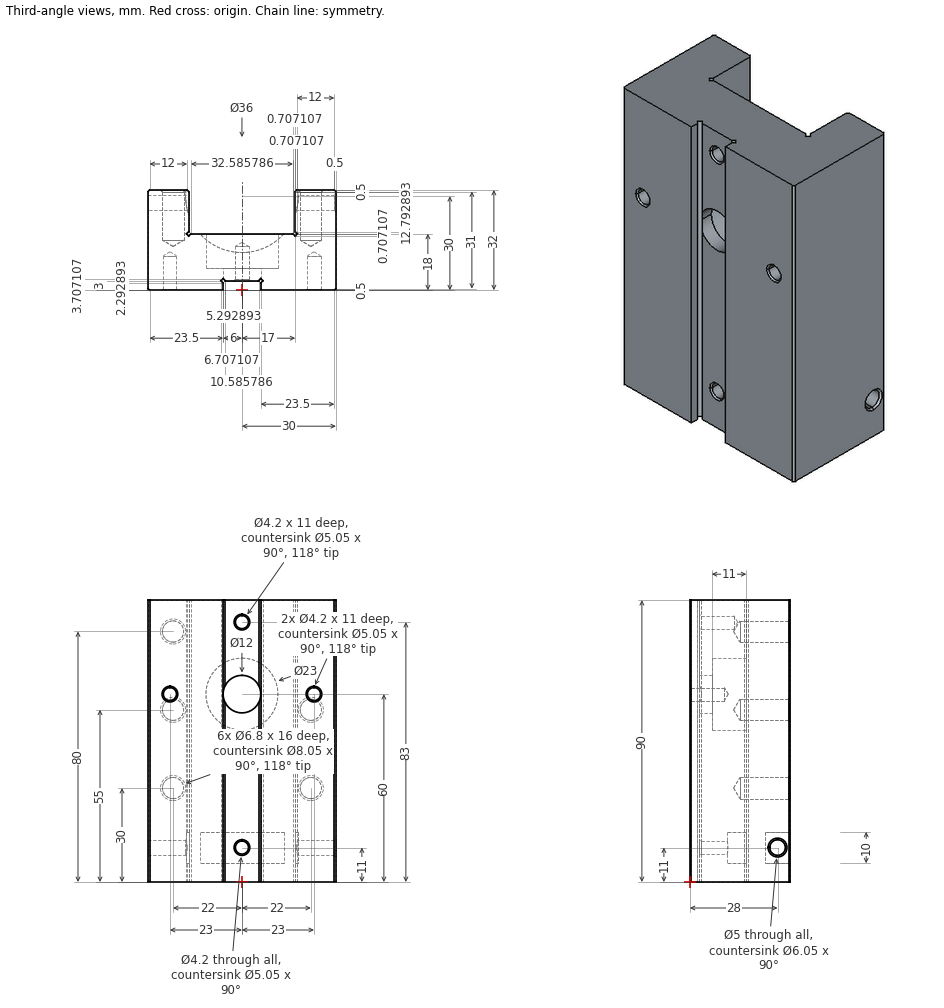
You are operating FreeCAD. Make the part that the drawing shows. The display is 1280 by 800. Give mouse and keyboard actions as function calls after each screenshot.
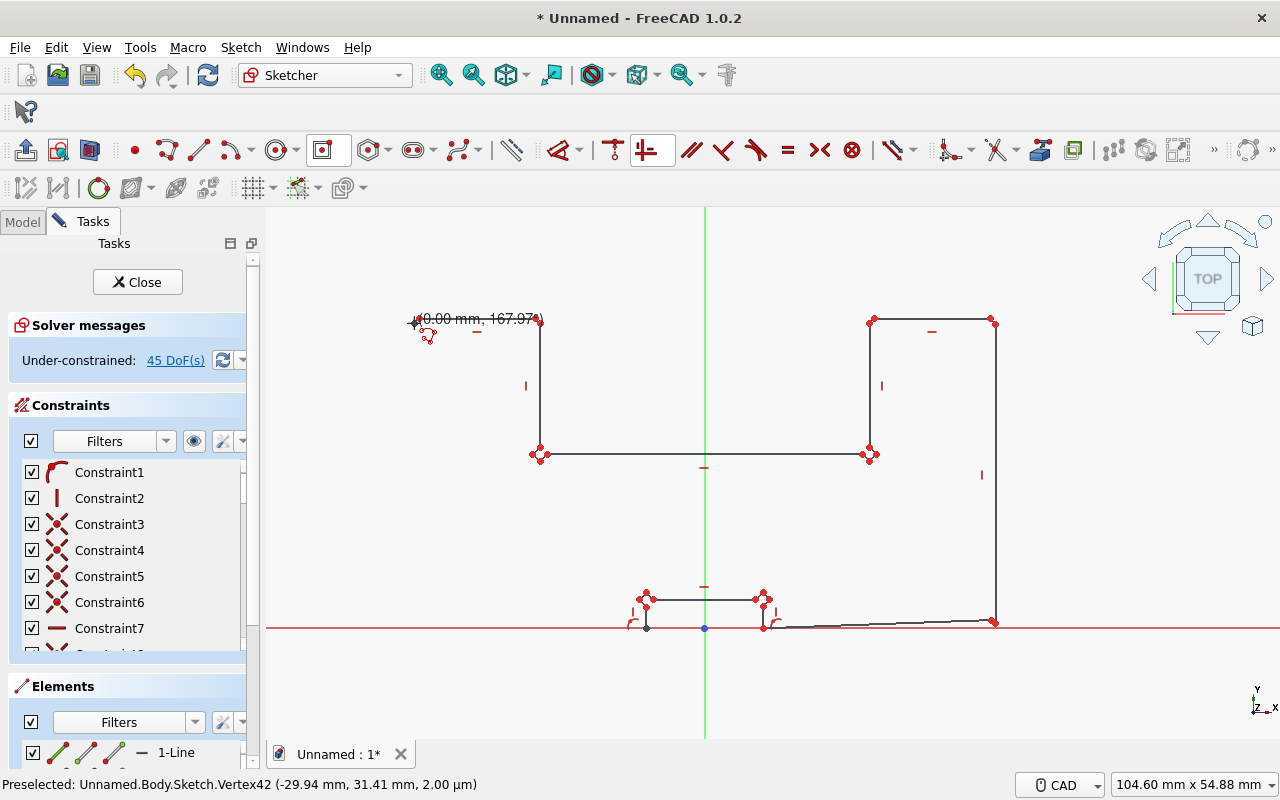
scroll(414, 623, up, 6)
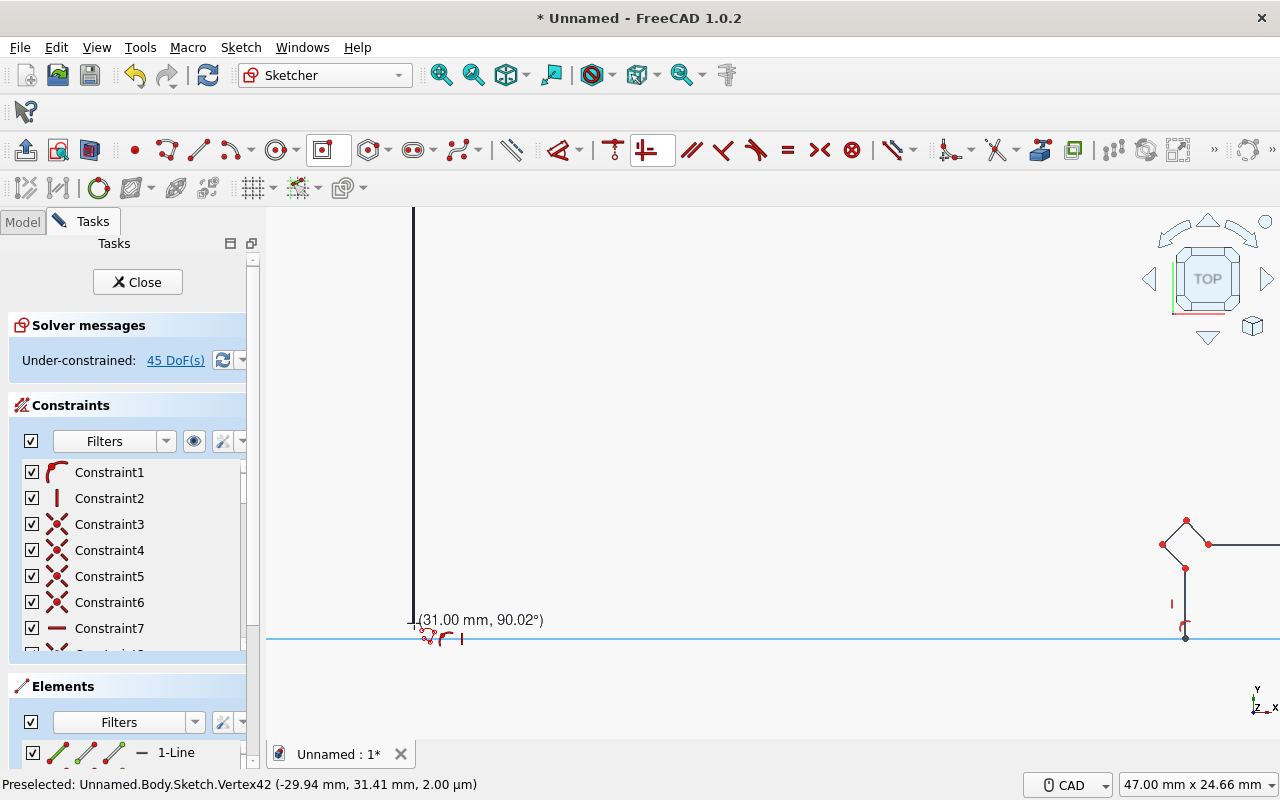
click(414, 623)
click(430, 630)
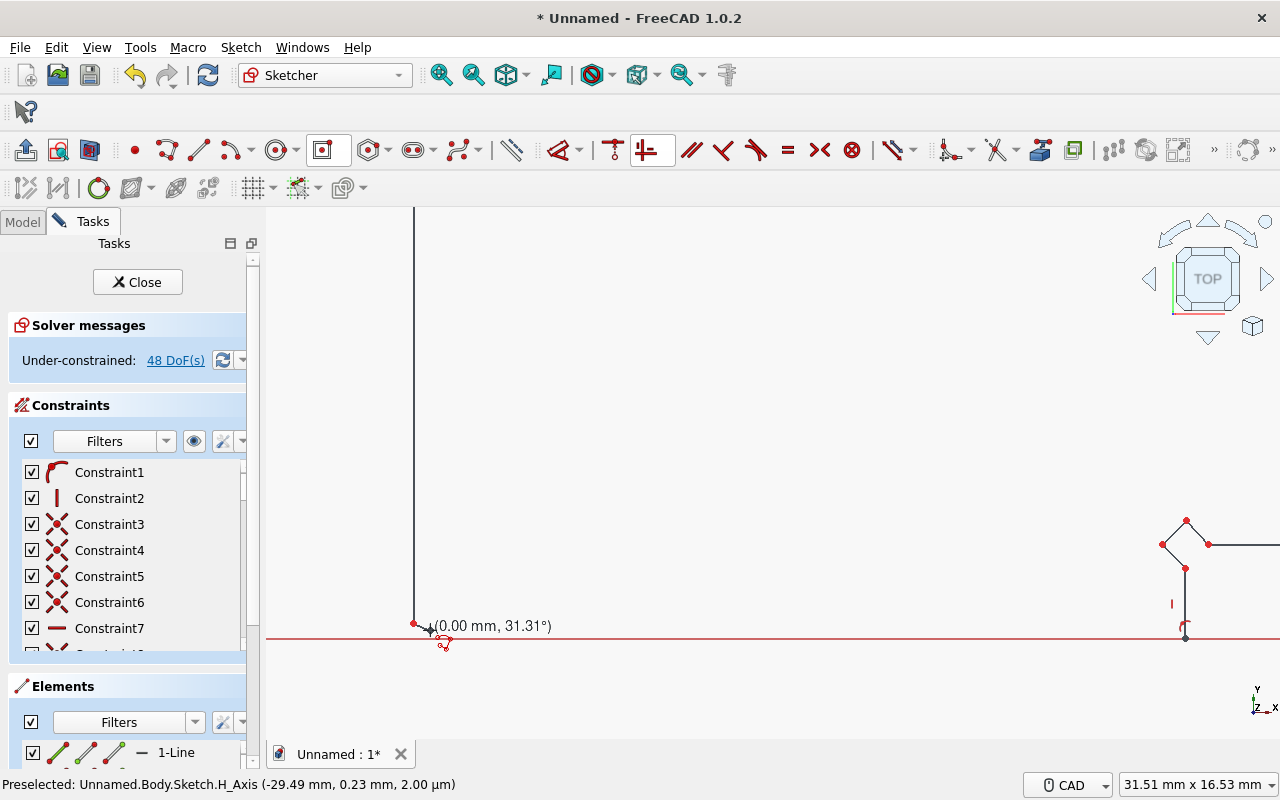
scroll(414, 623, down, 6)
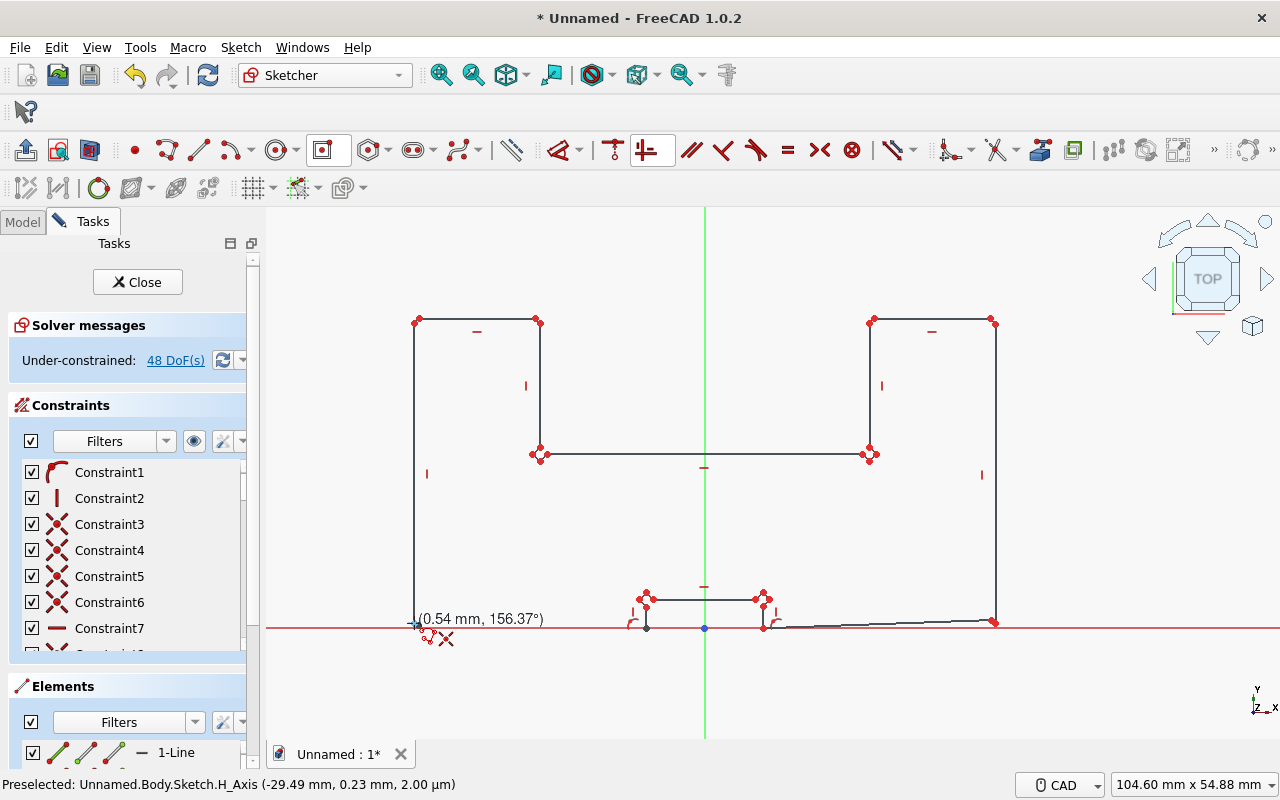
scroll(647, 628, up, 2)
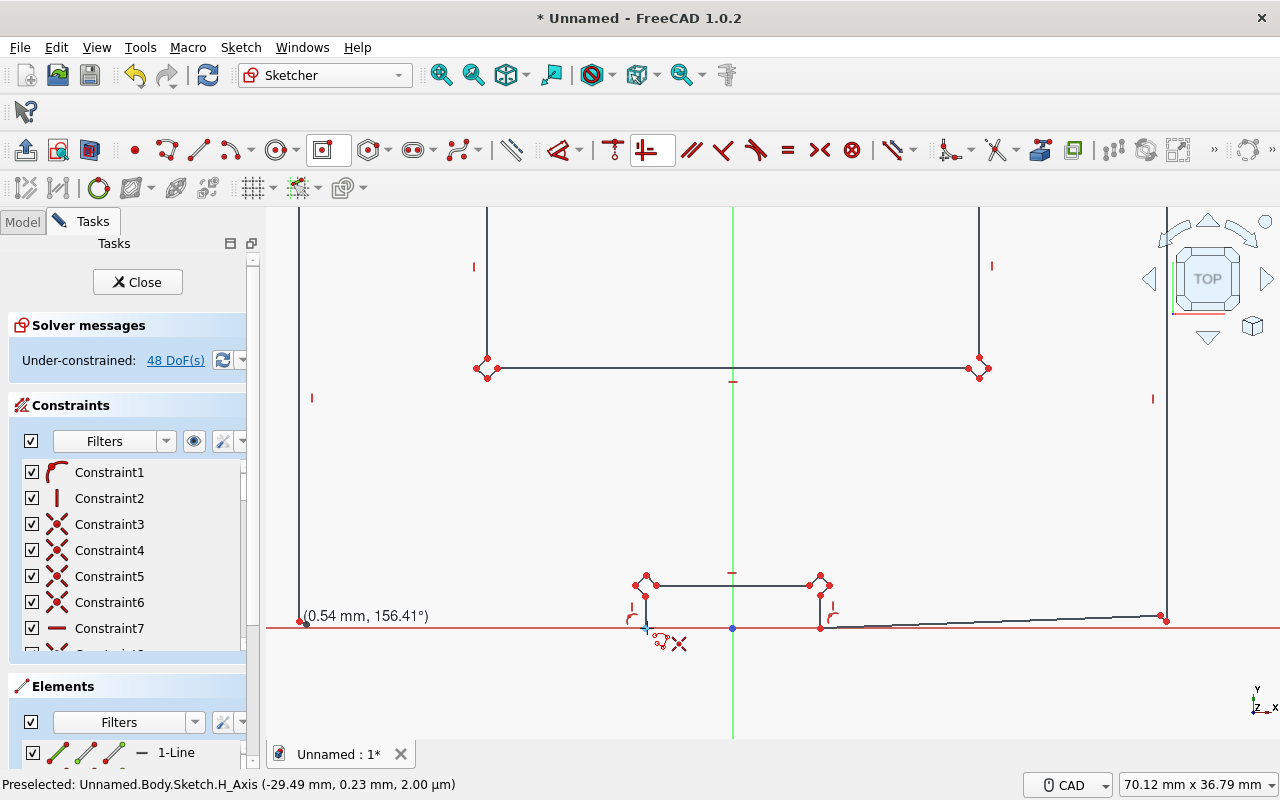
click(646, 628)
key(Escape)
key(Escape)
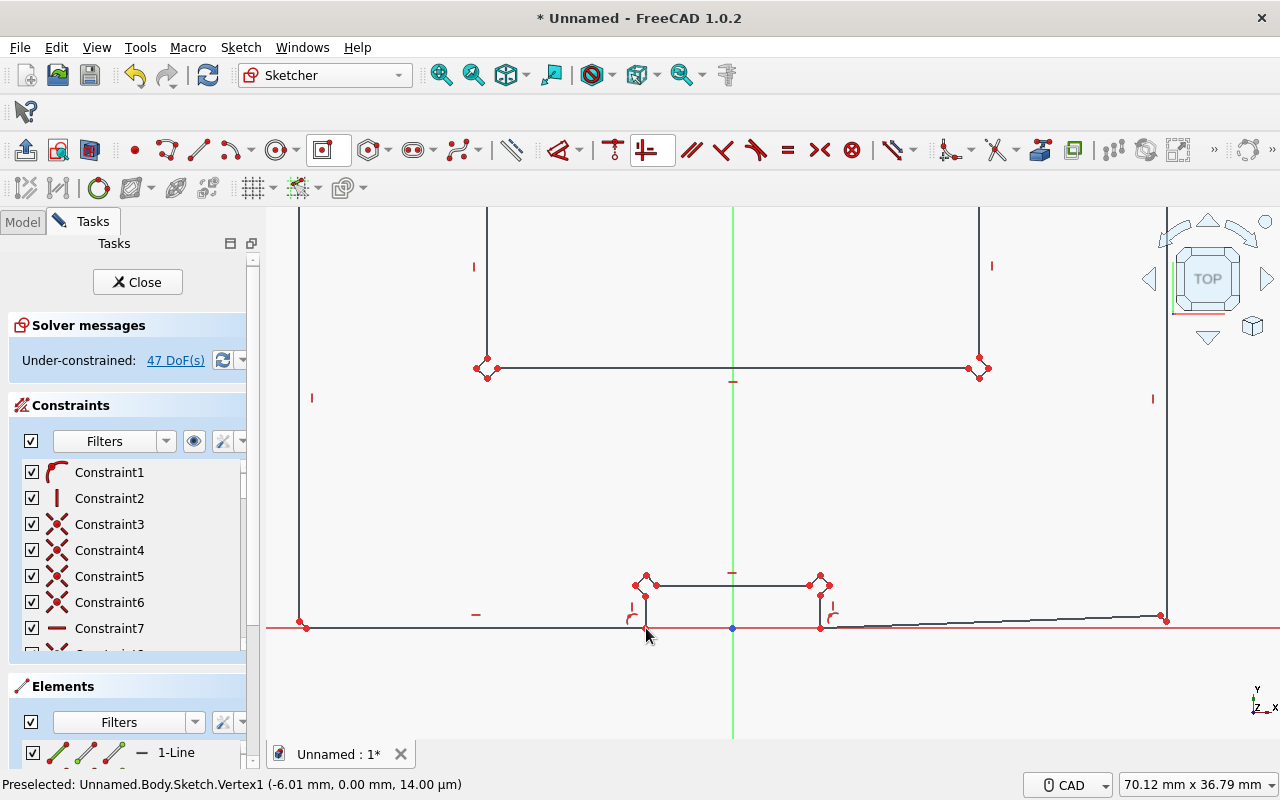
click(922, 624)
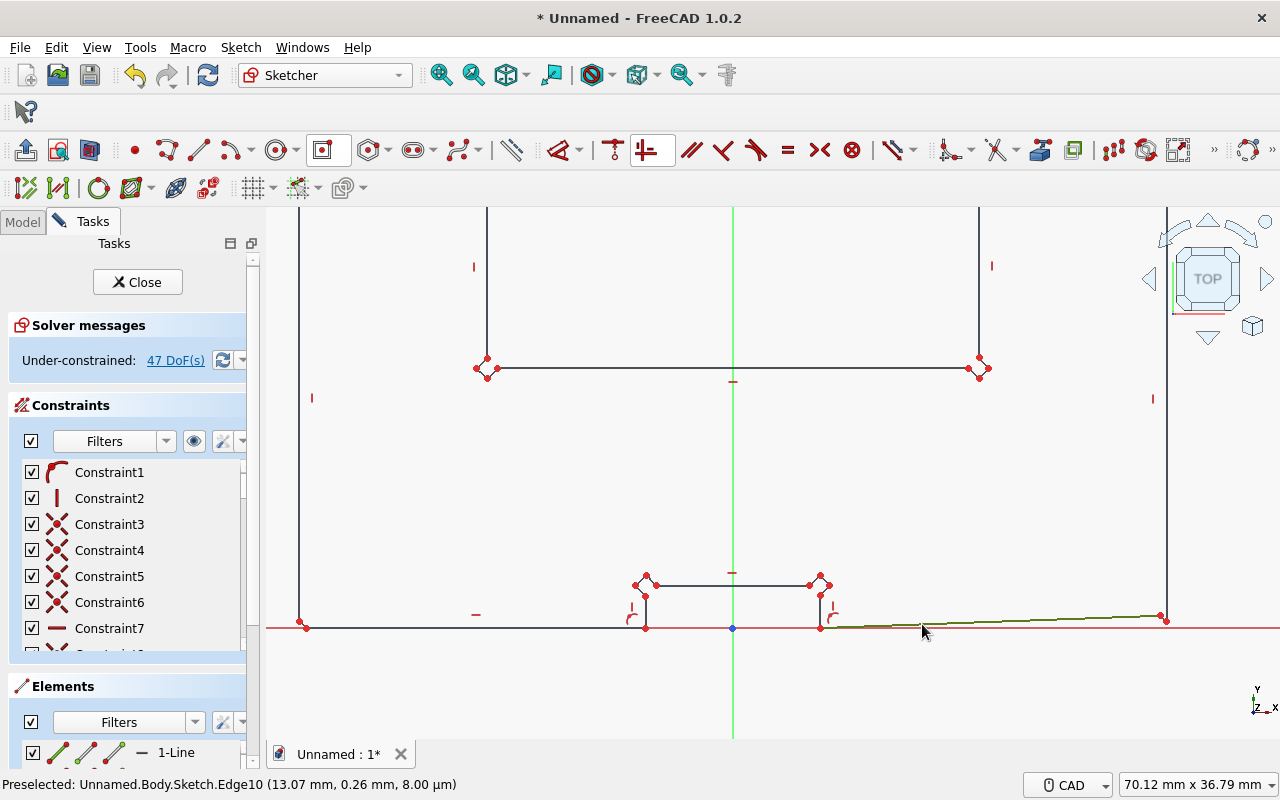
key(h)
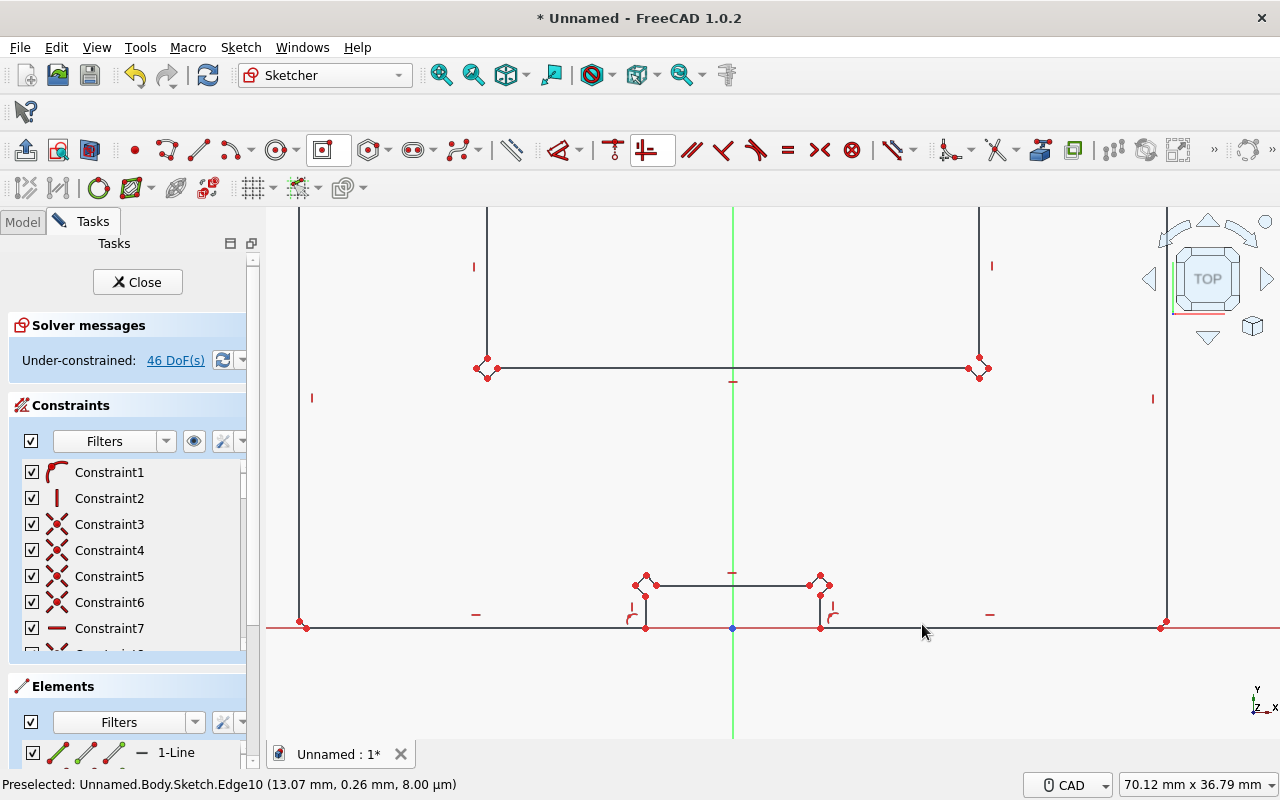
click(646, 575)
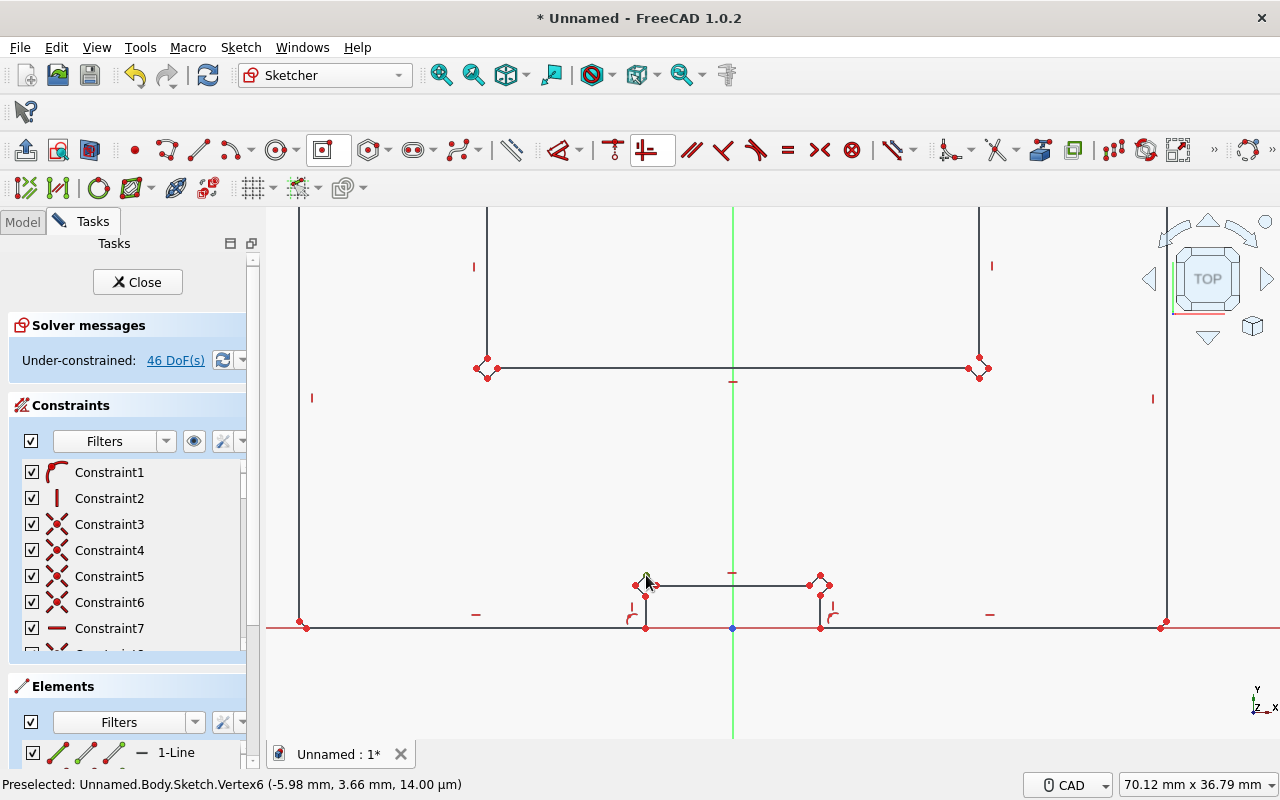
click(820, 575)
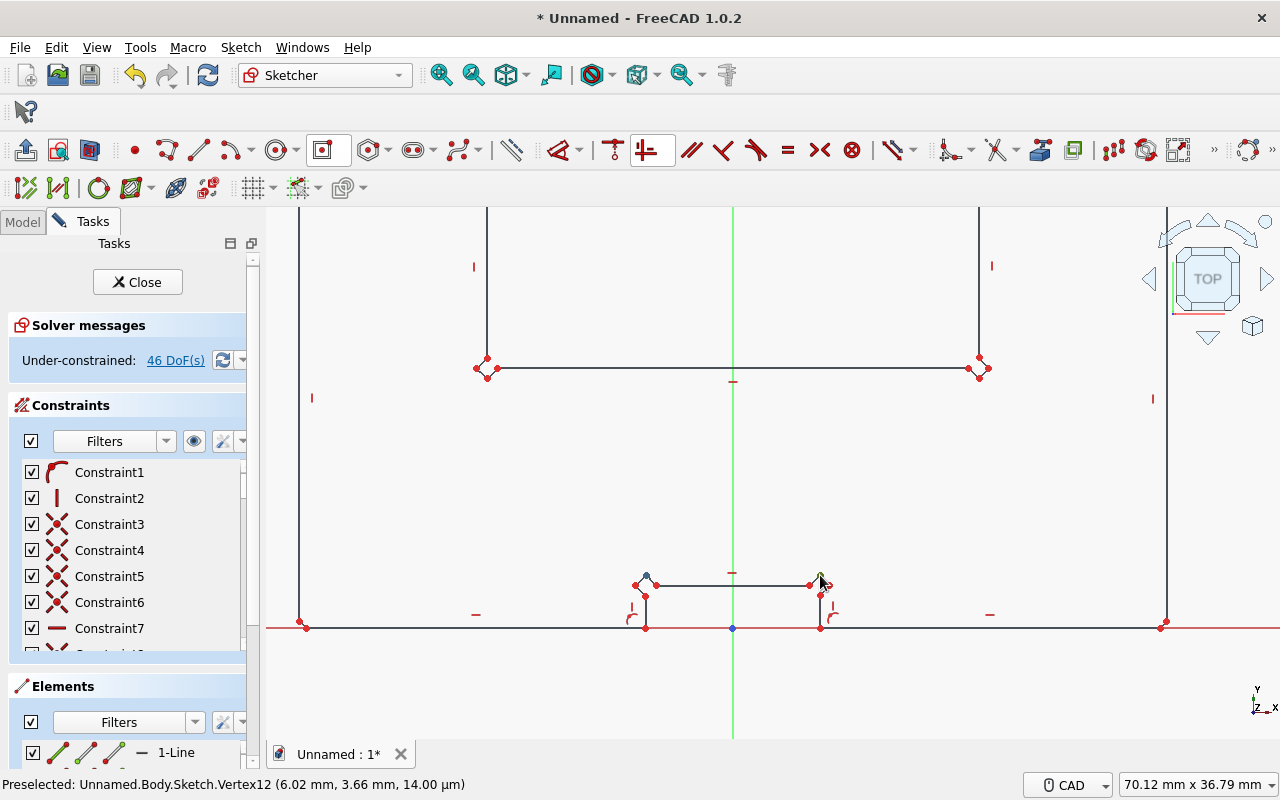
click(733, 677)